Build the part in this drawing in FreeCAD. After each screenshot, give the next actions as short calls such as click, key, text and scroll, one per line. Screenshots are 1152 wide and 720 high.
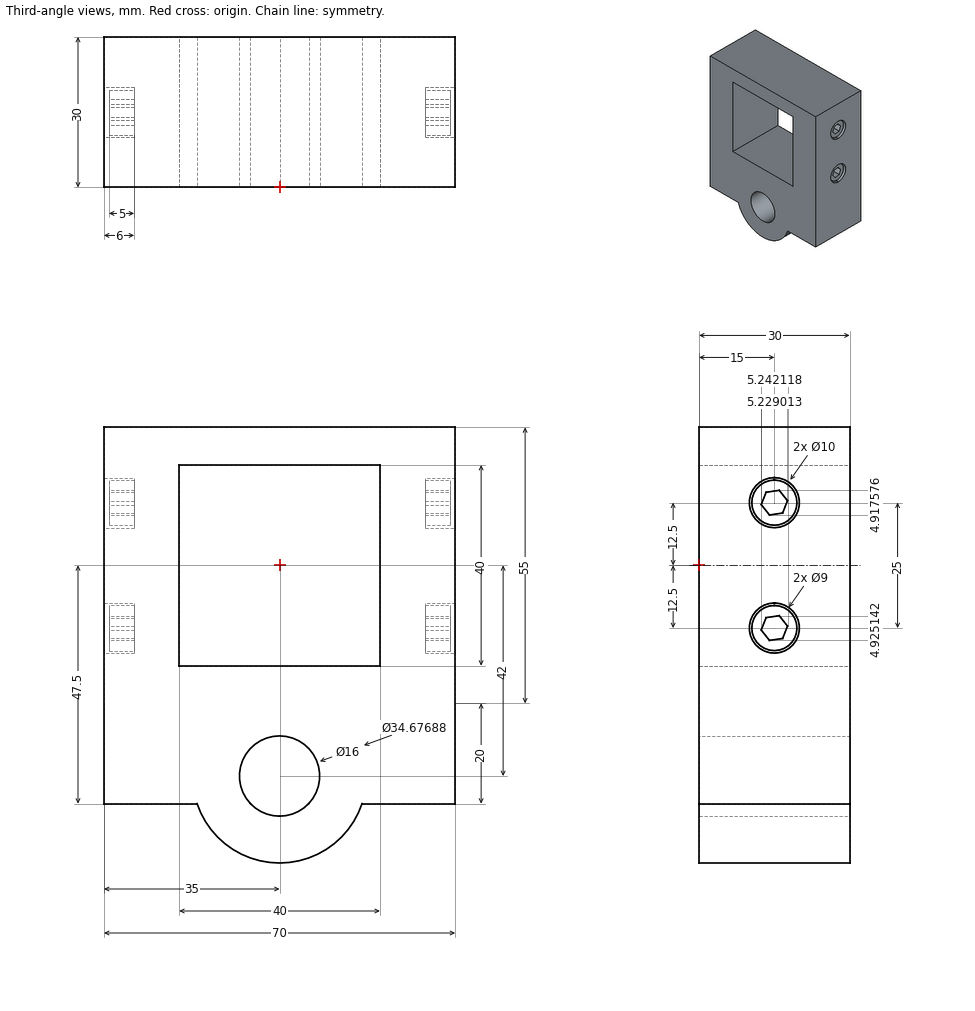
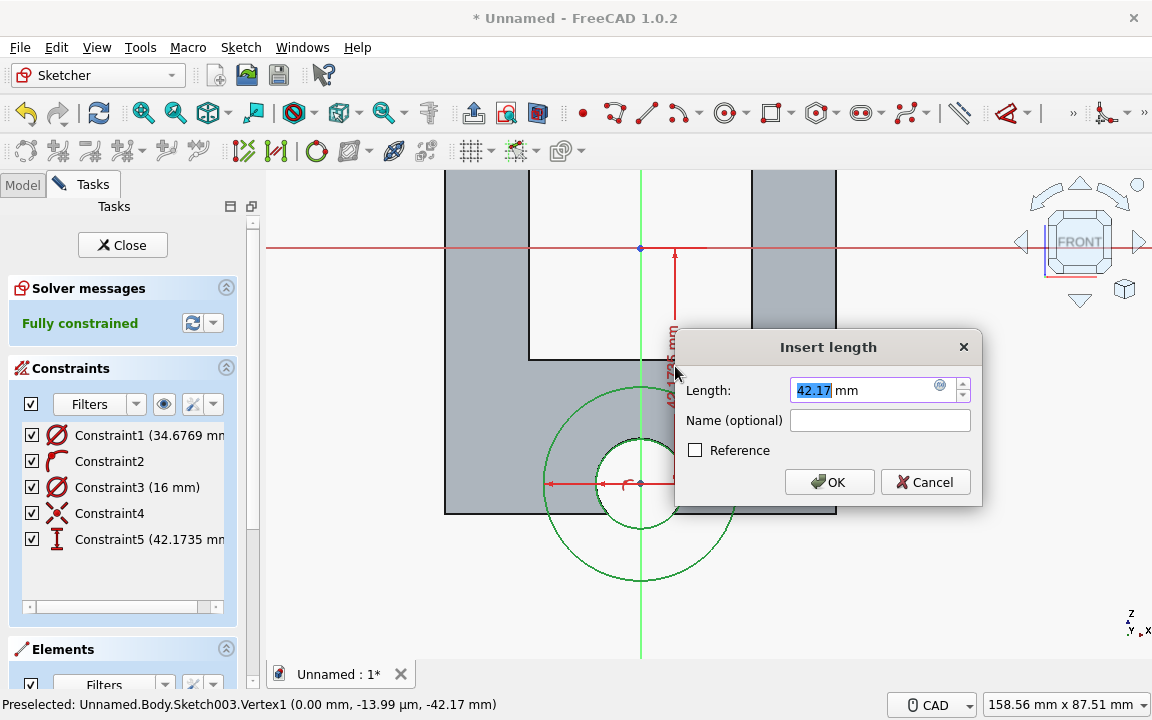
text(42)
key(Return)
key(Escape)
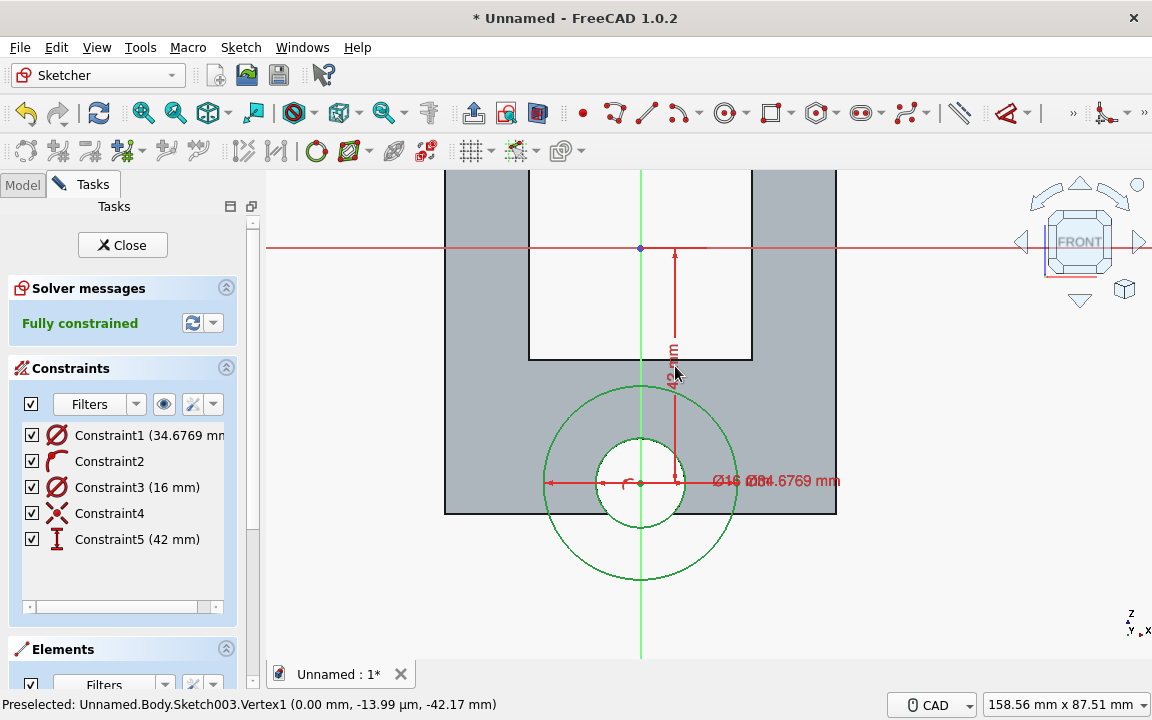
click(123, 245)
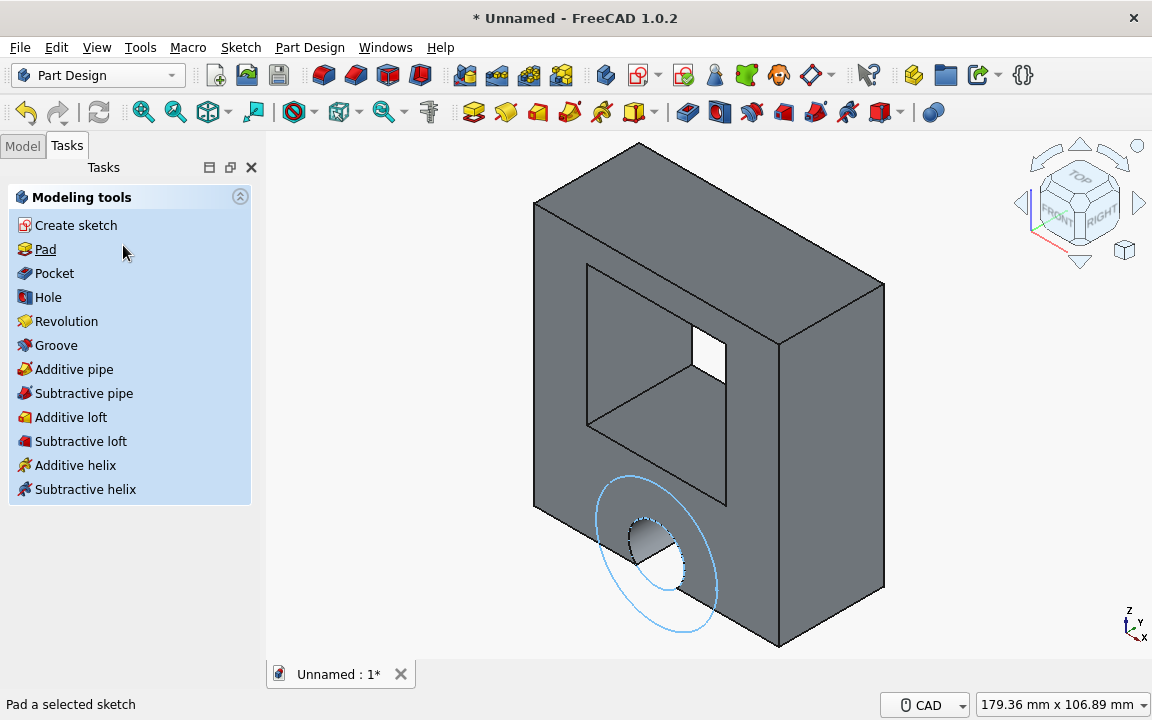
click(474, 112)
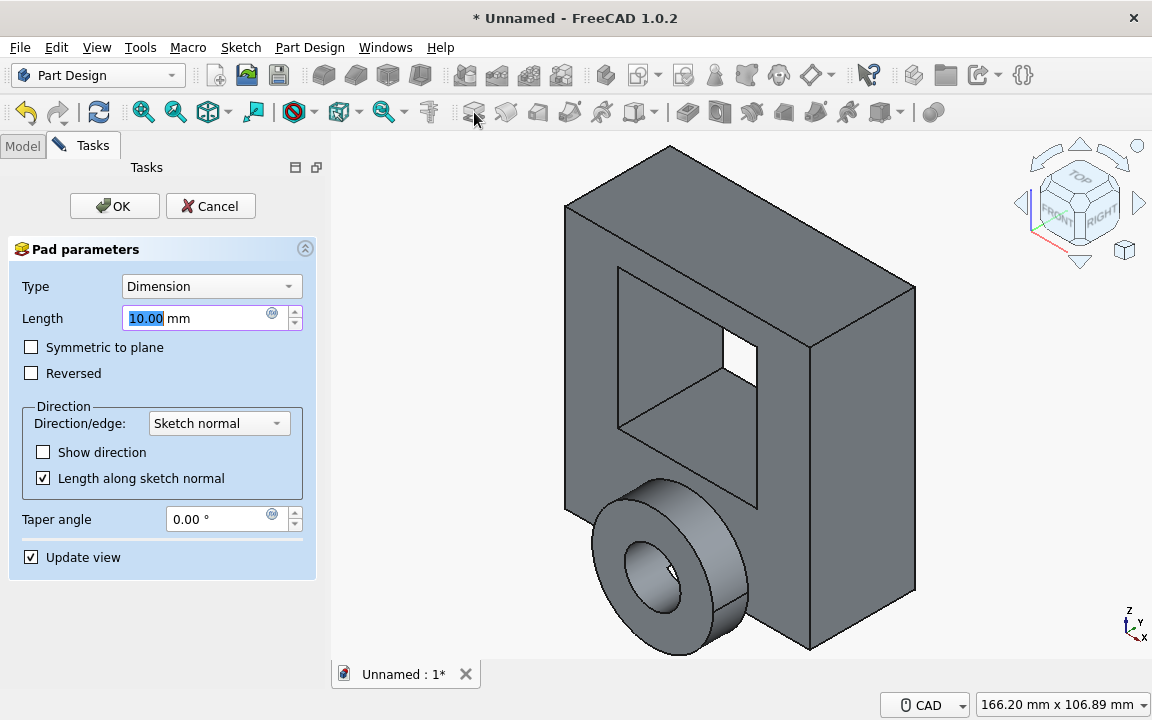
text(30)
key(Tab)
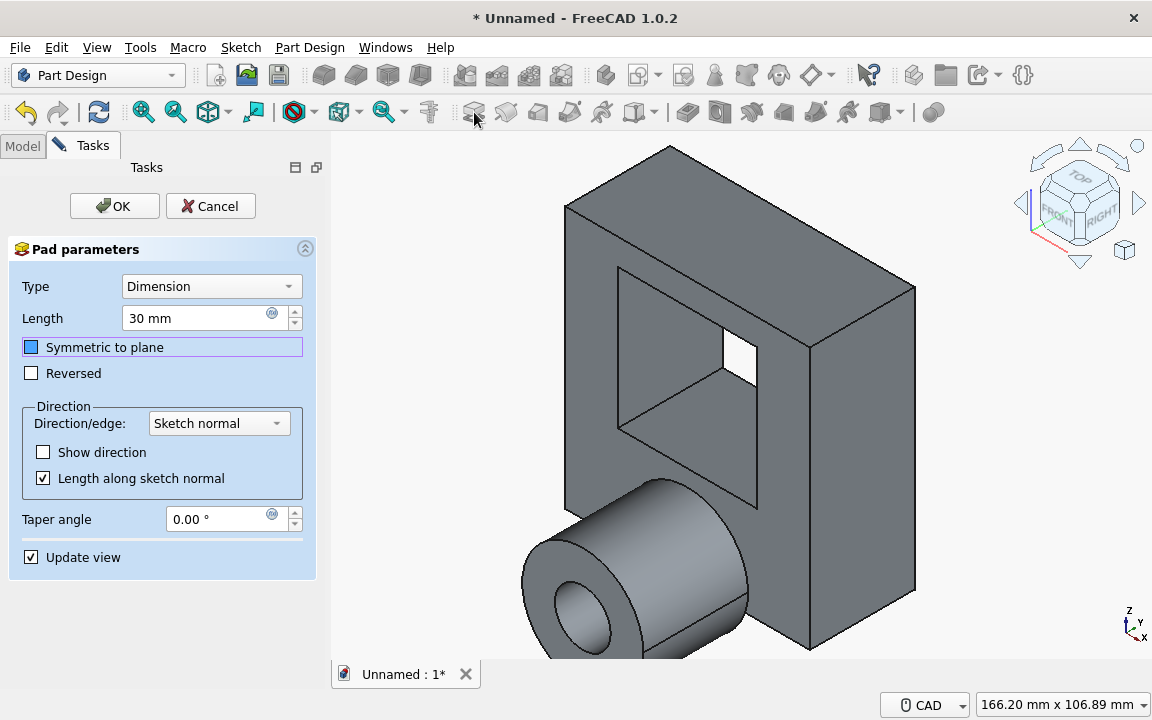
click(30, 373)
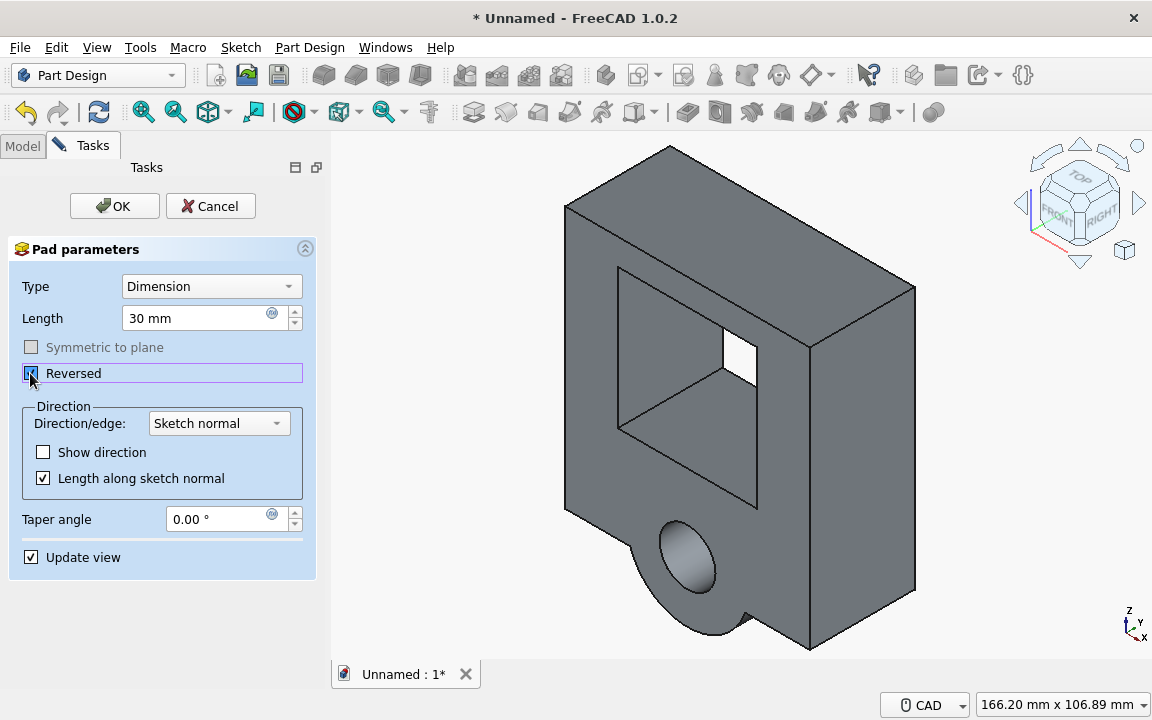
click(115, 206)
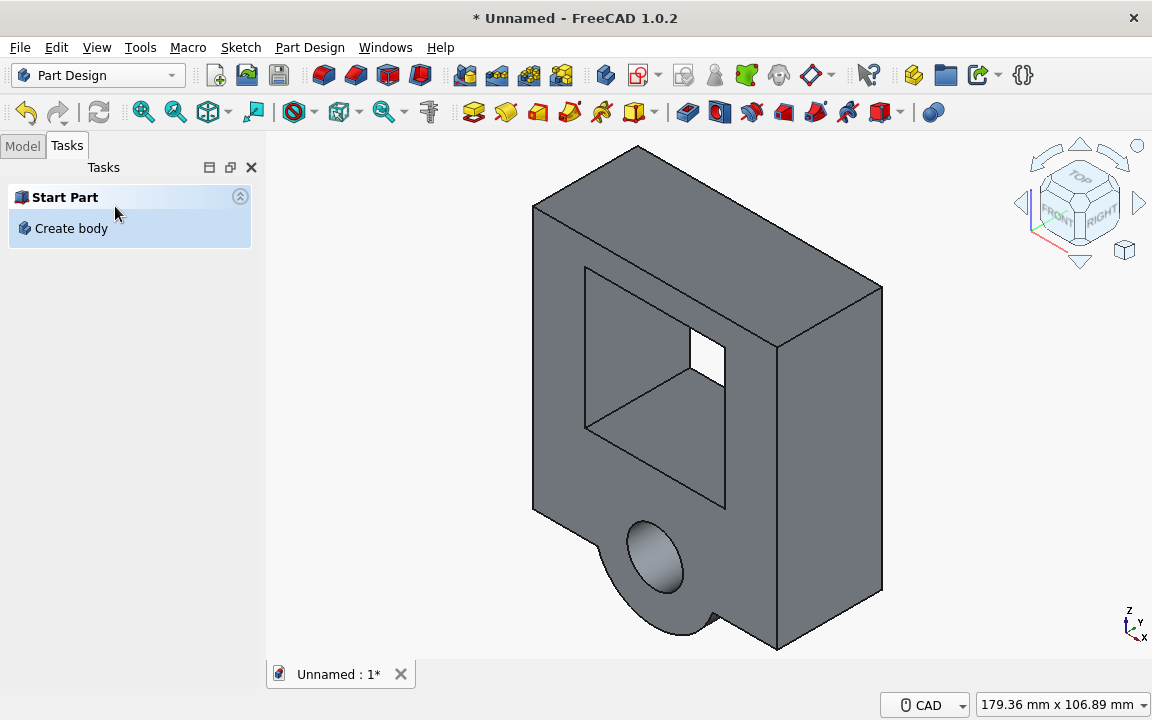
click(144, 112)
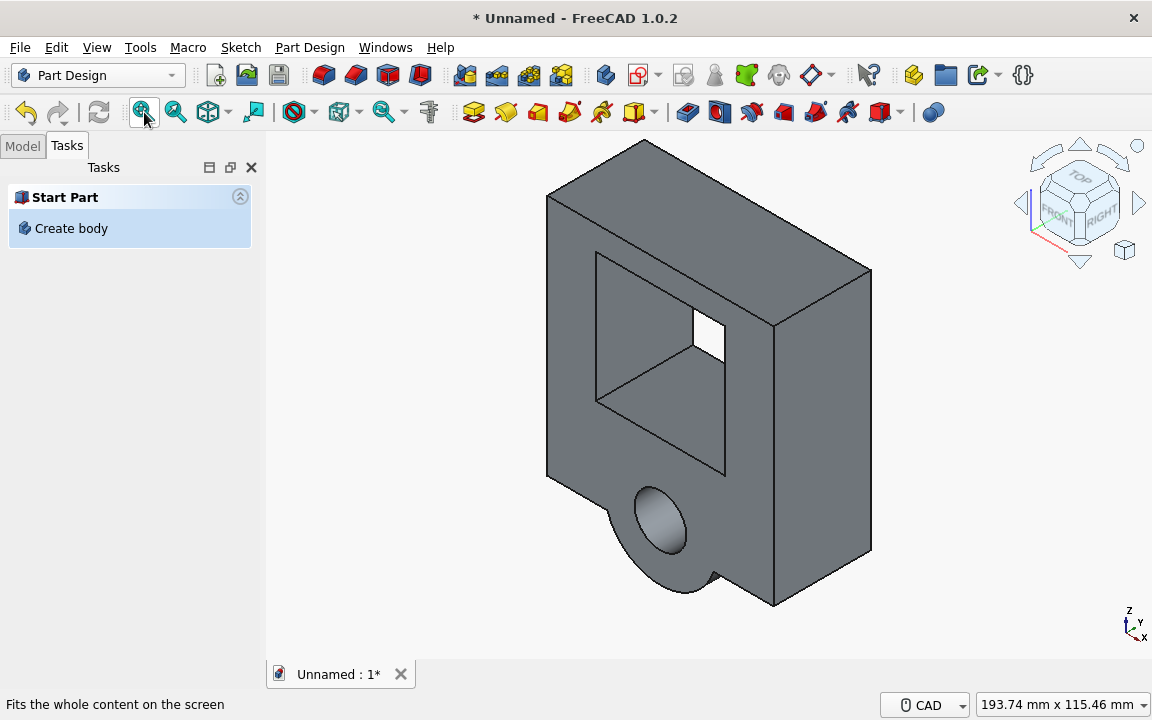
key(6)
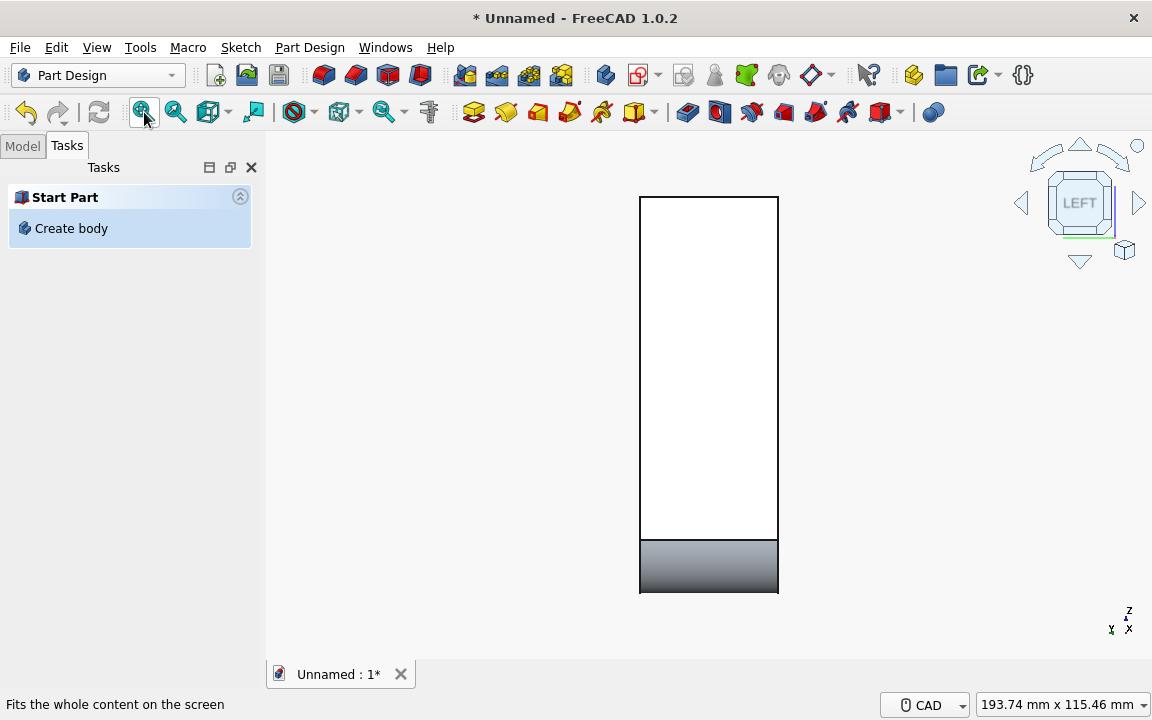
click(709, 465)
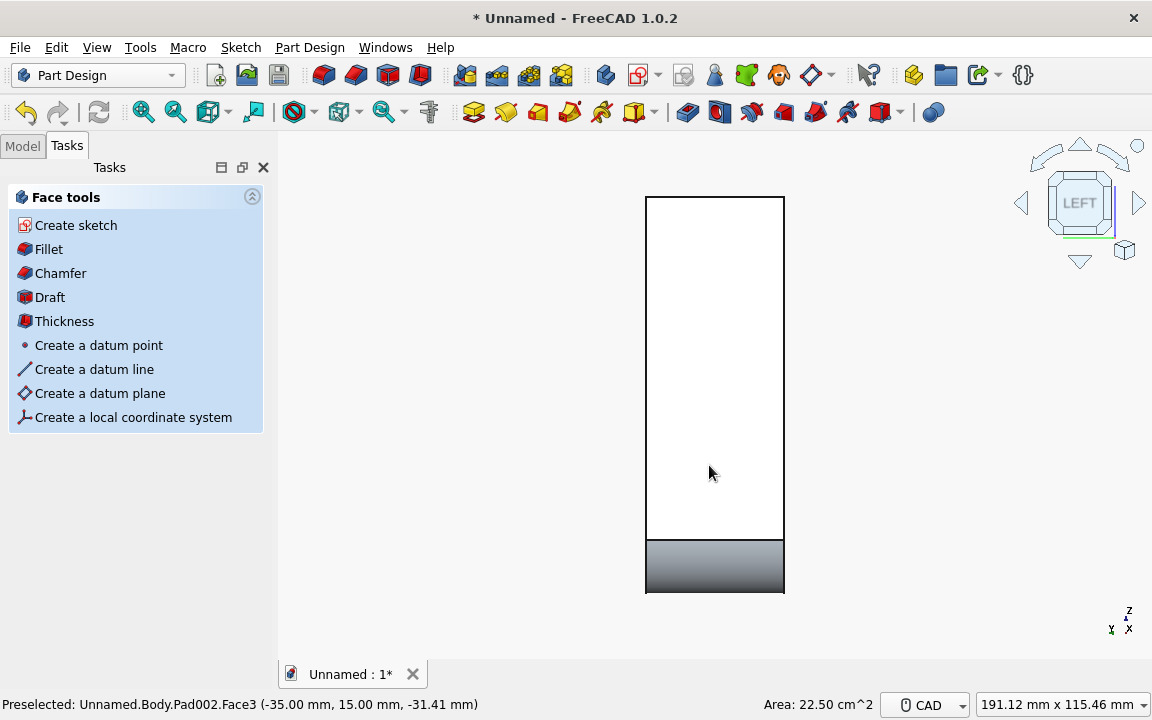
click(638, 76)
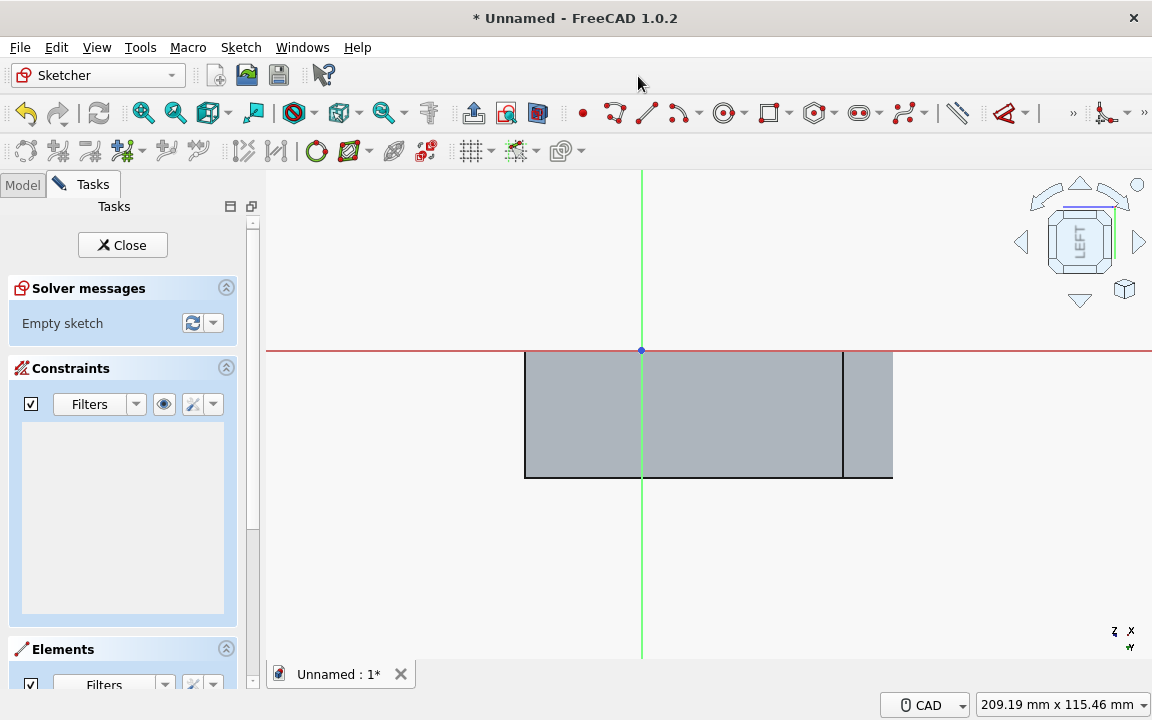
scroll(642, 384, up, 6)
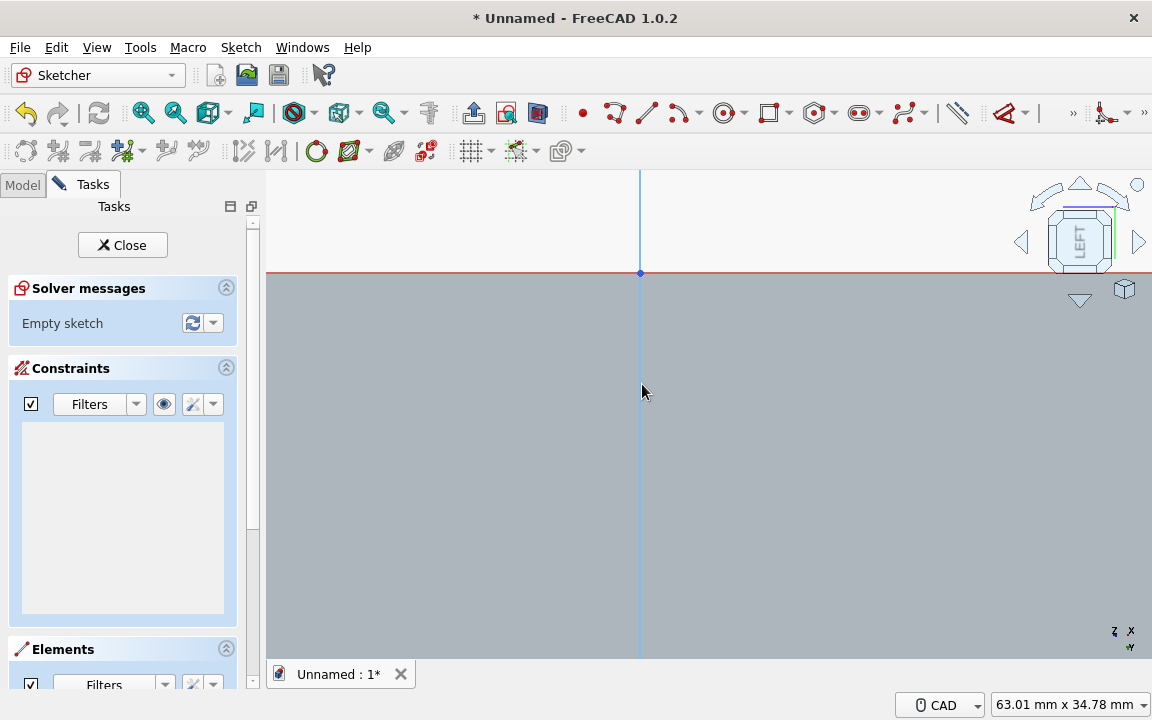
click(724, 114)